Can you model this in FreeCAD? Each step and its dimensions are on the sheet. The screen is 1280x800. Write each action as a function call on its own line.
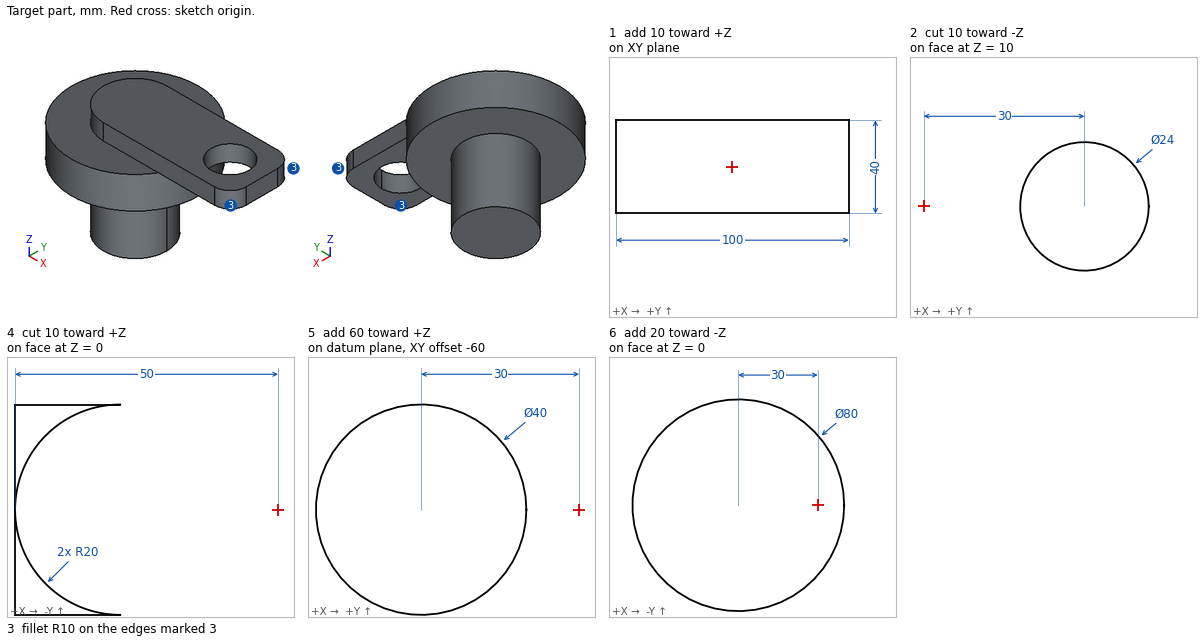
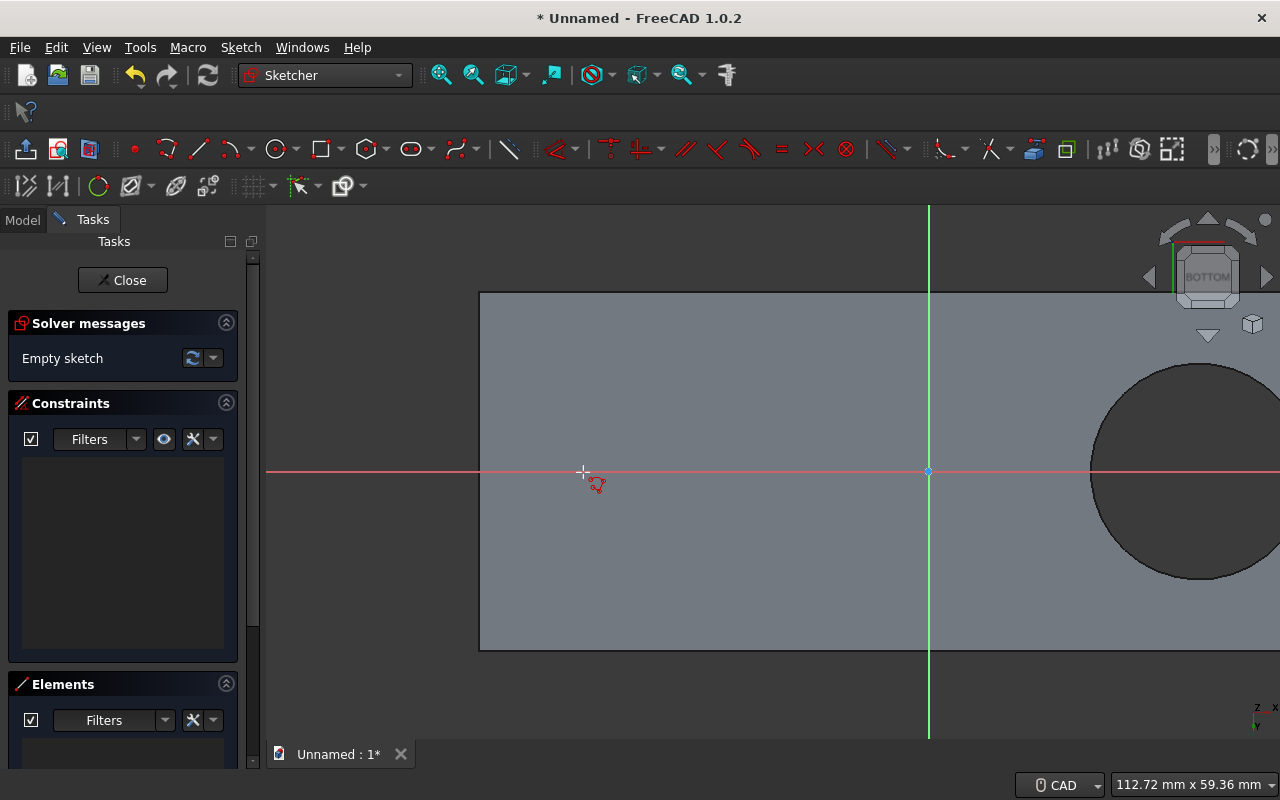
click(479, 472)
click(479, 651)
click(659, 651)
right_click(659, 651)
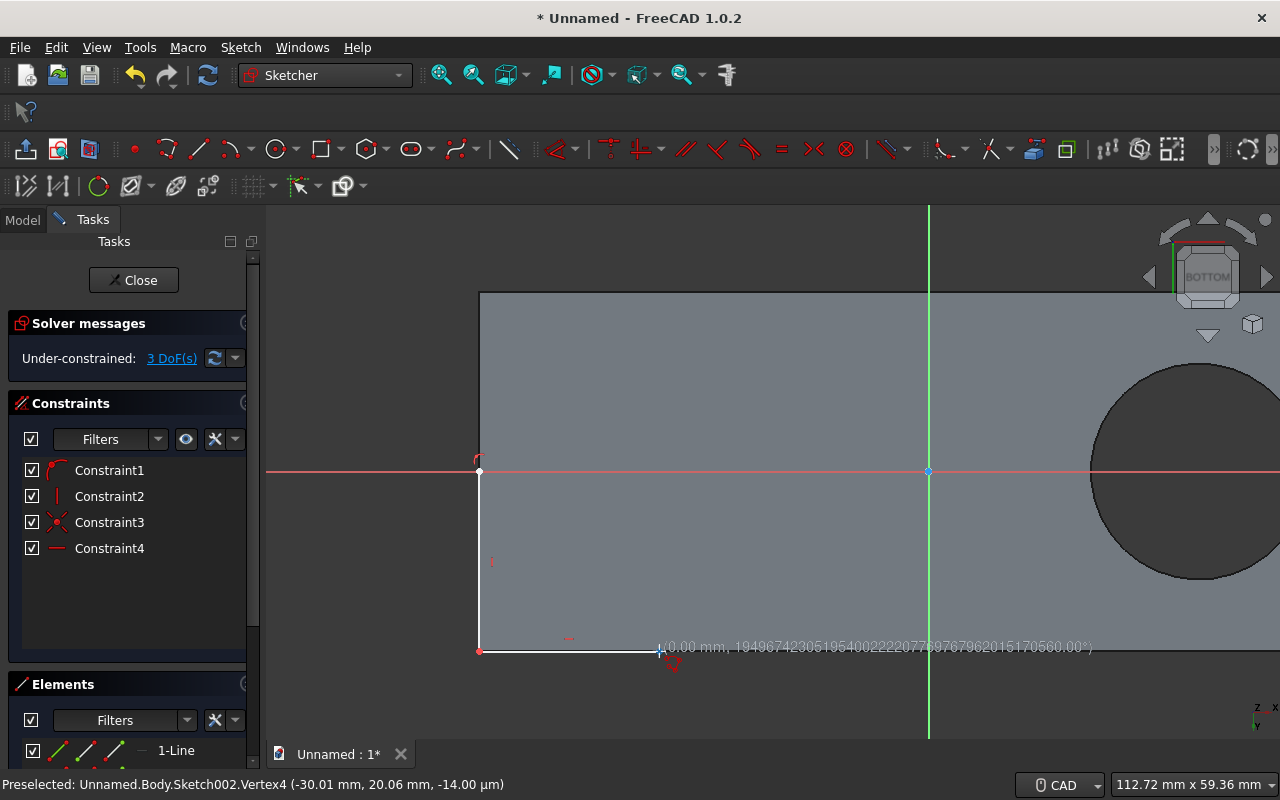
key(g)
key(3)
key(a)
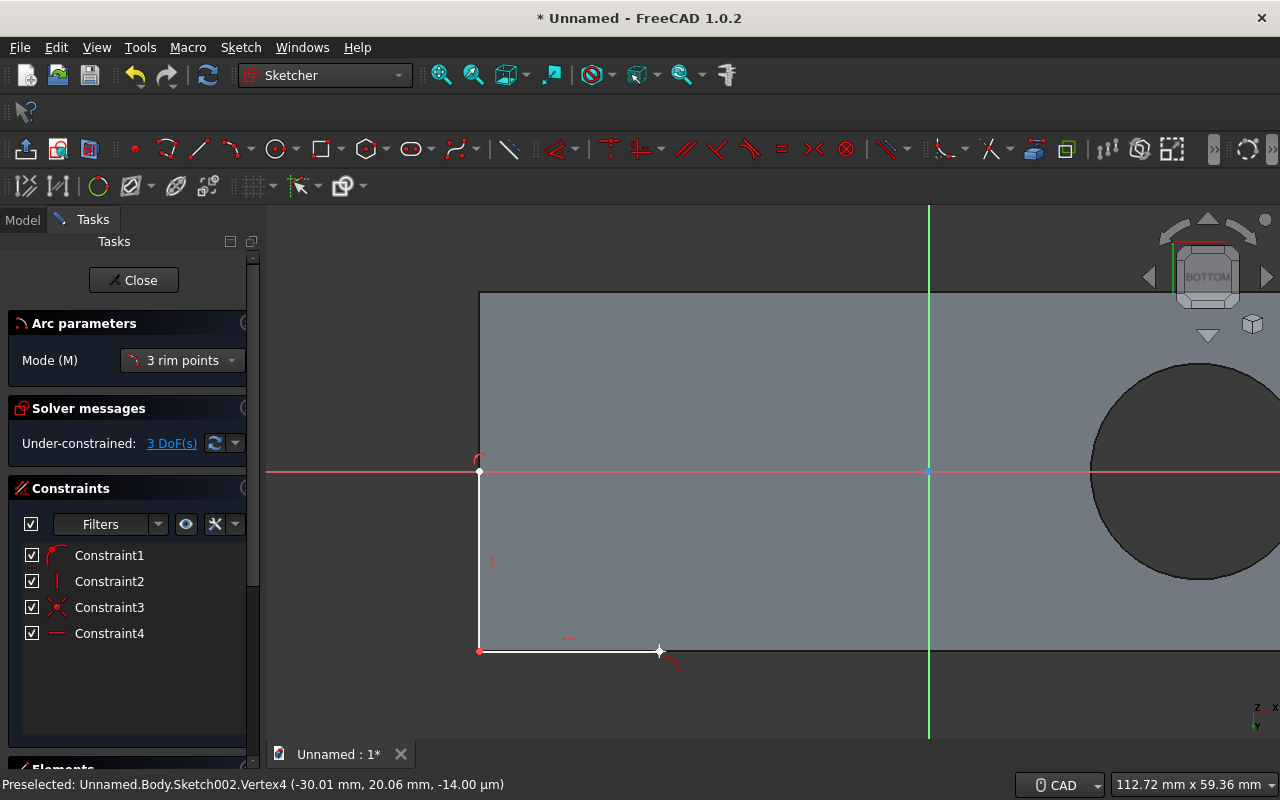
click(659, 652)
click(479, 472)
click(532, 599)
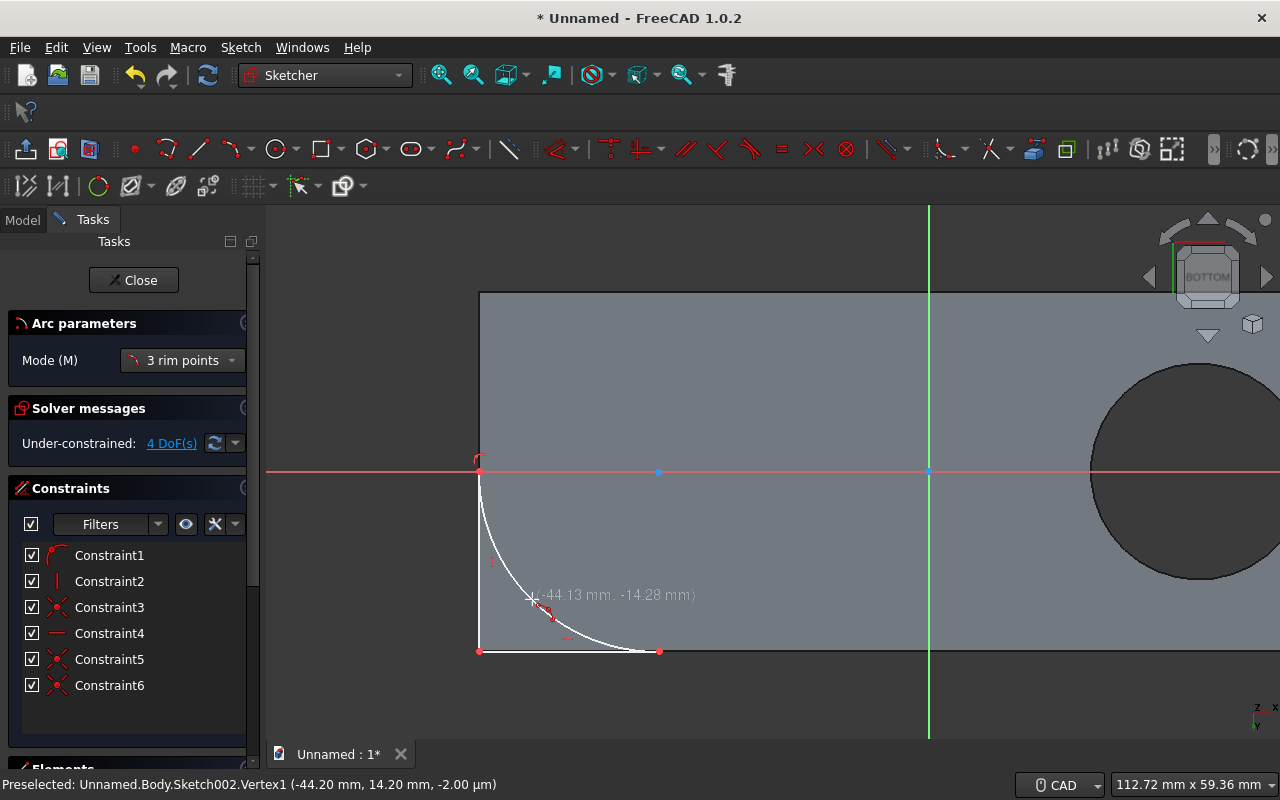
click(168, 150)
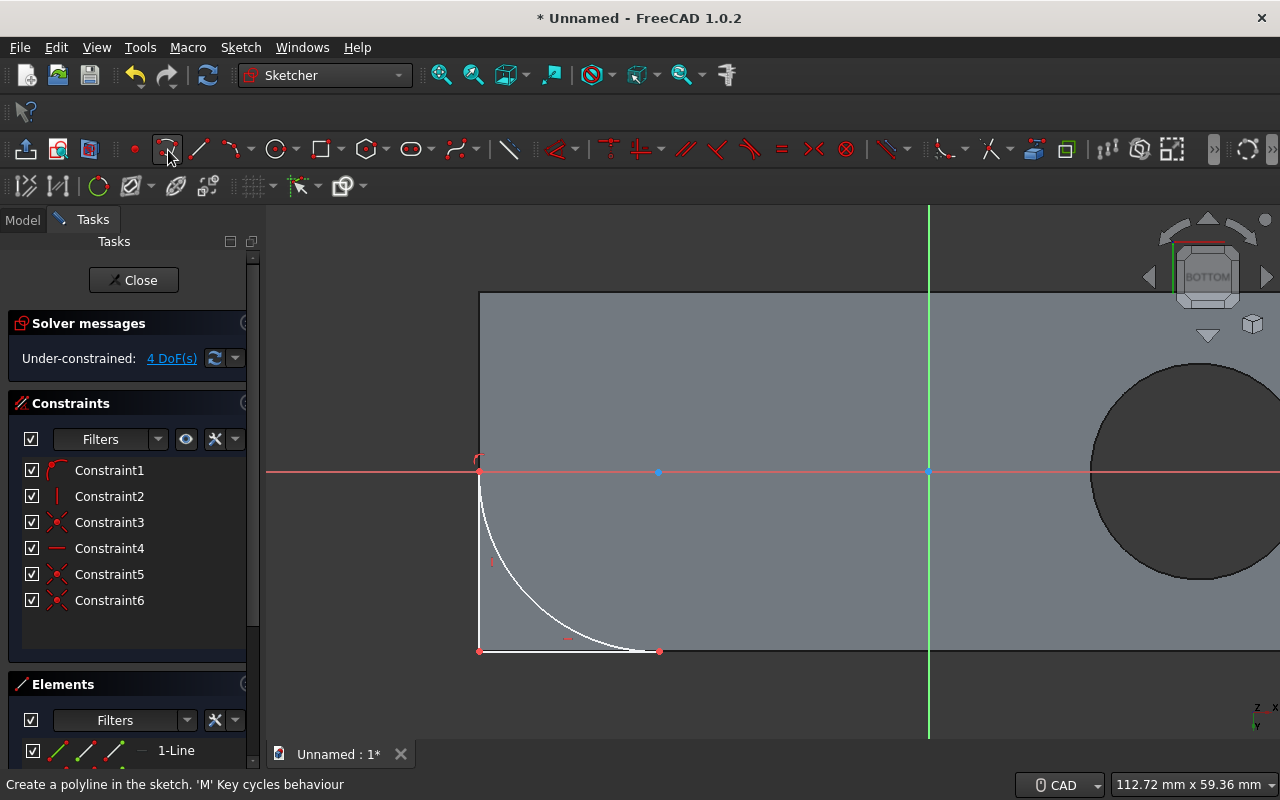
click(659, 292)
click(479, 292)
click(479, 472)
right_click(479, 292)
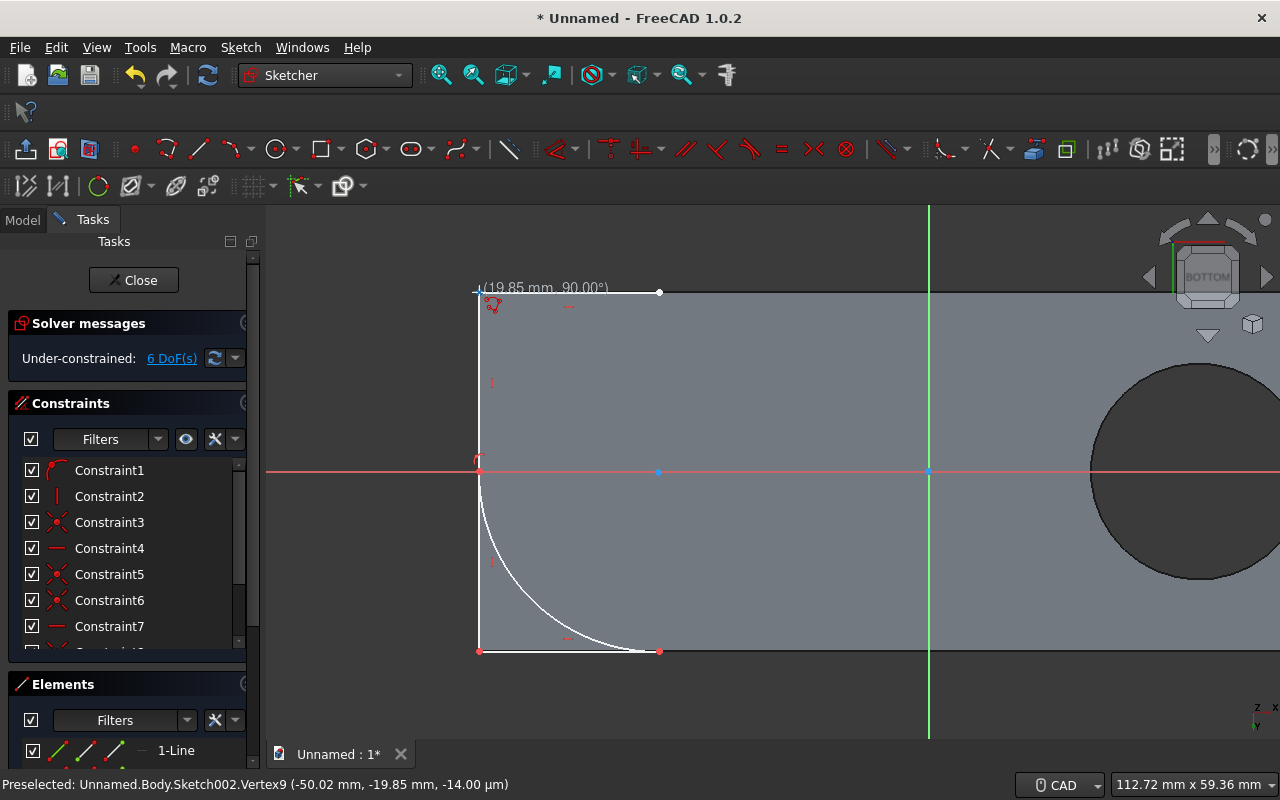
click(232, 150)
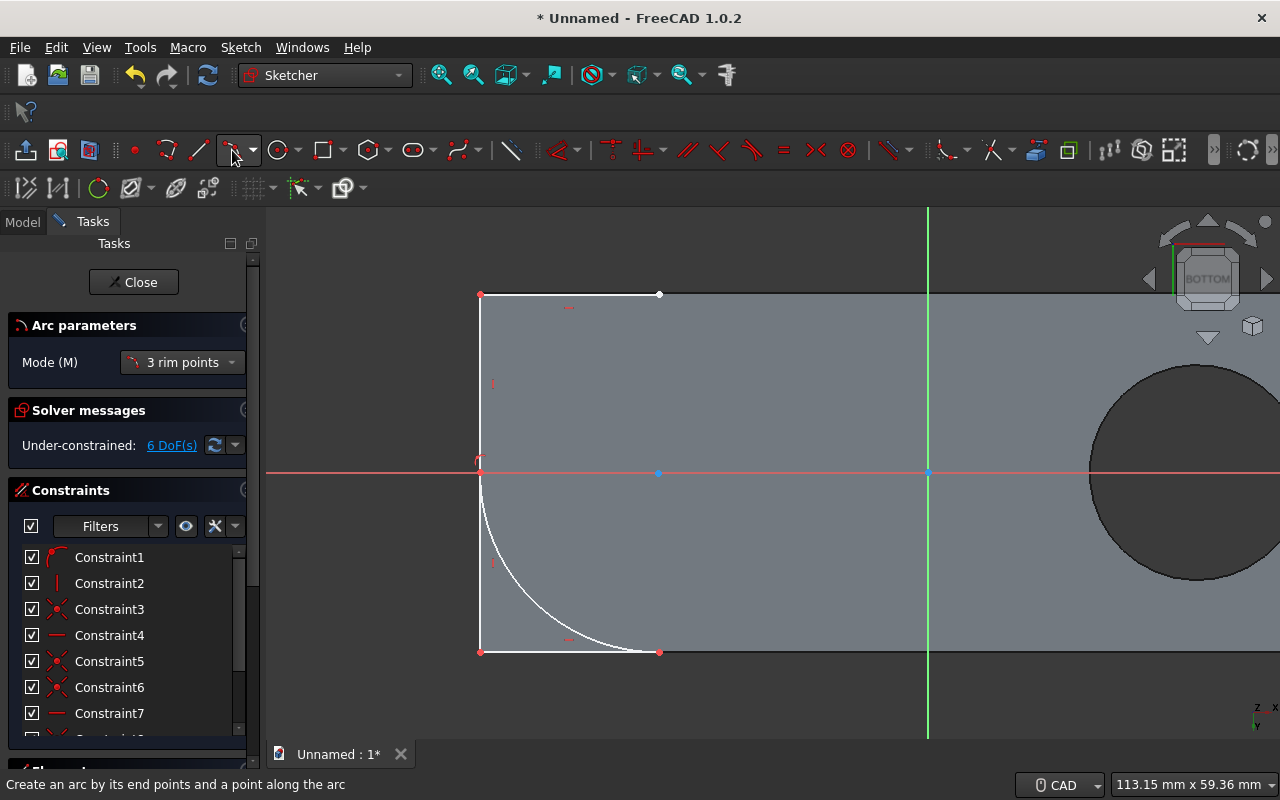
click(480, 473)
click(659, 295)
click(533, 346)
key(Escape)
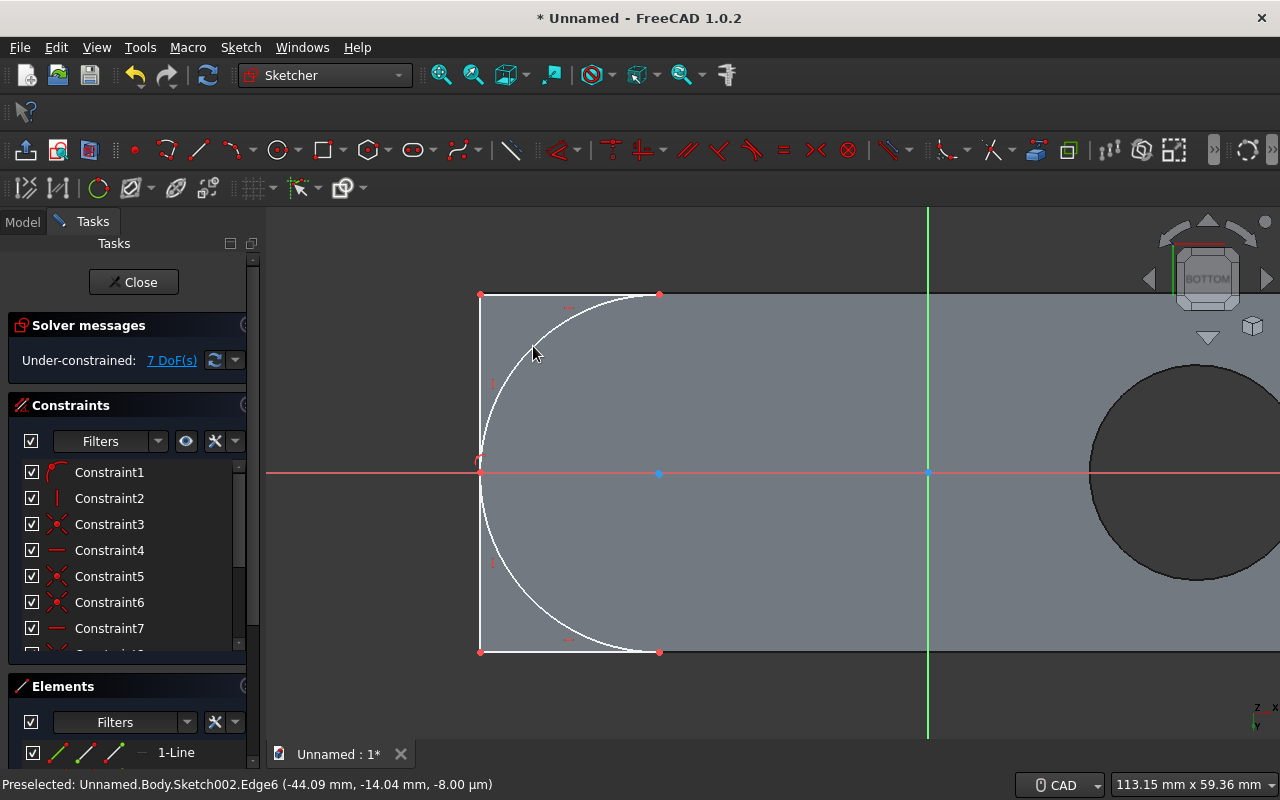
click(480, 598)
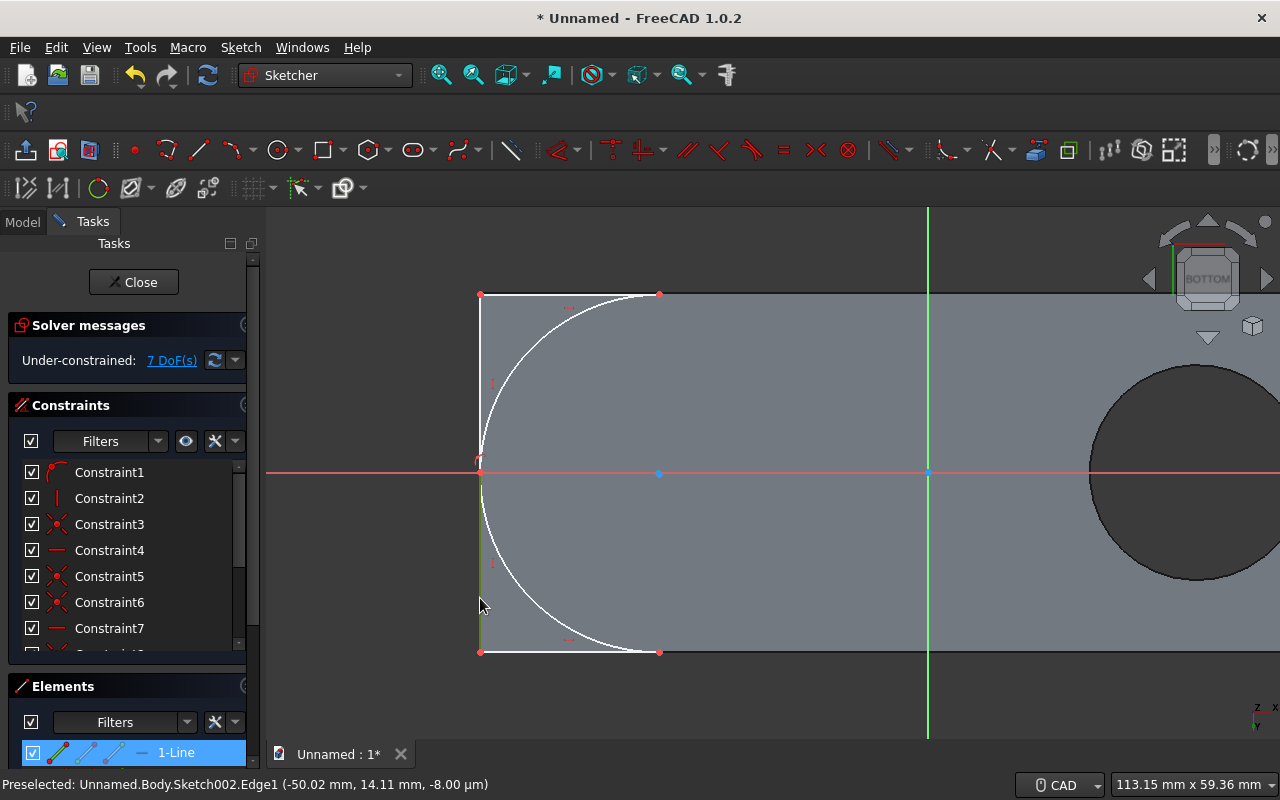
click(499, 554)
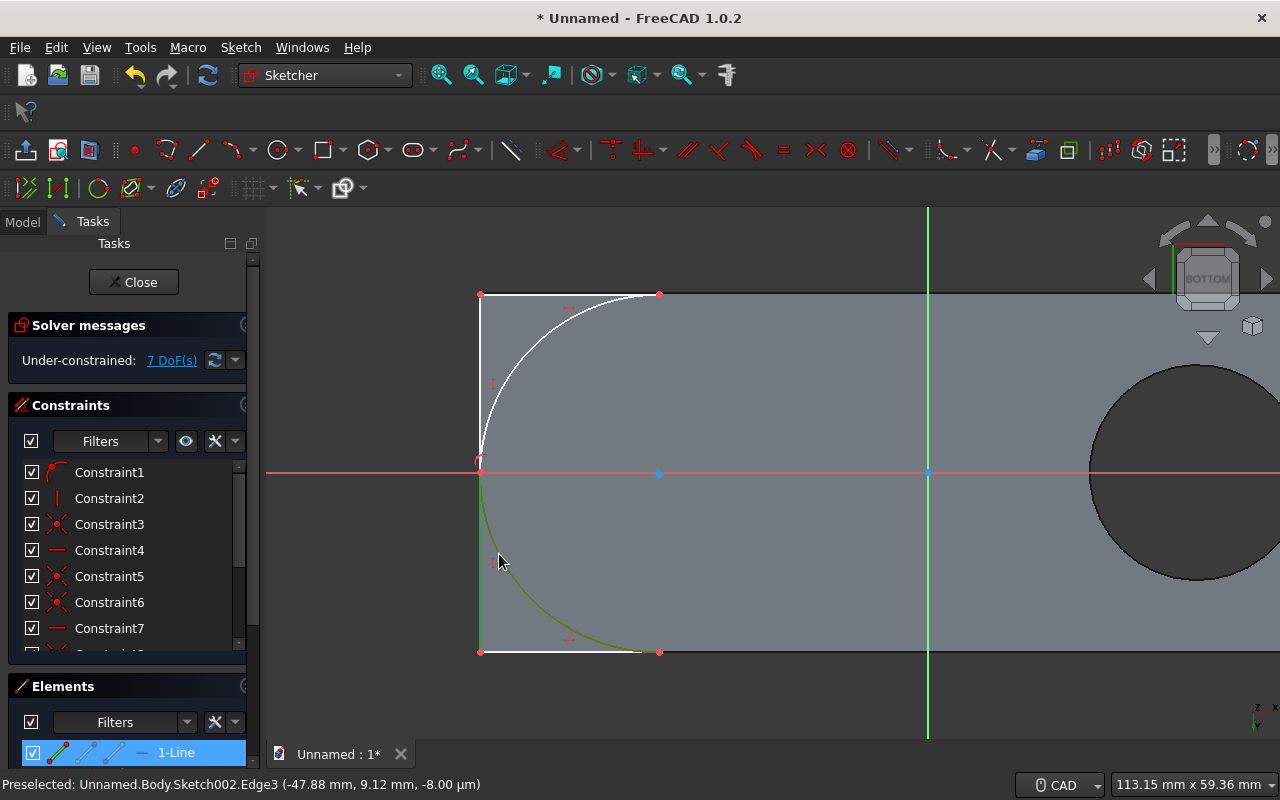
key(t)